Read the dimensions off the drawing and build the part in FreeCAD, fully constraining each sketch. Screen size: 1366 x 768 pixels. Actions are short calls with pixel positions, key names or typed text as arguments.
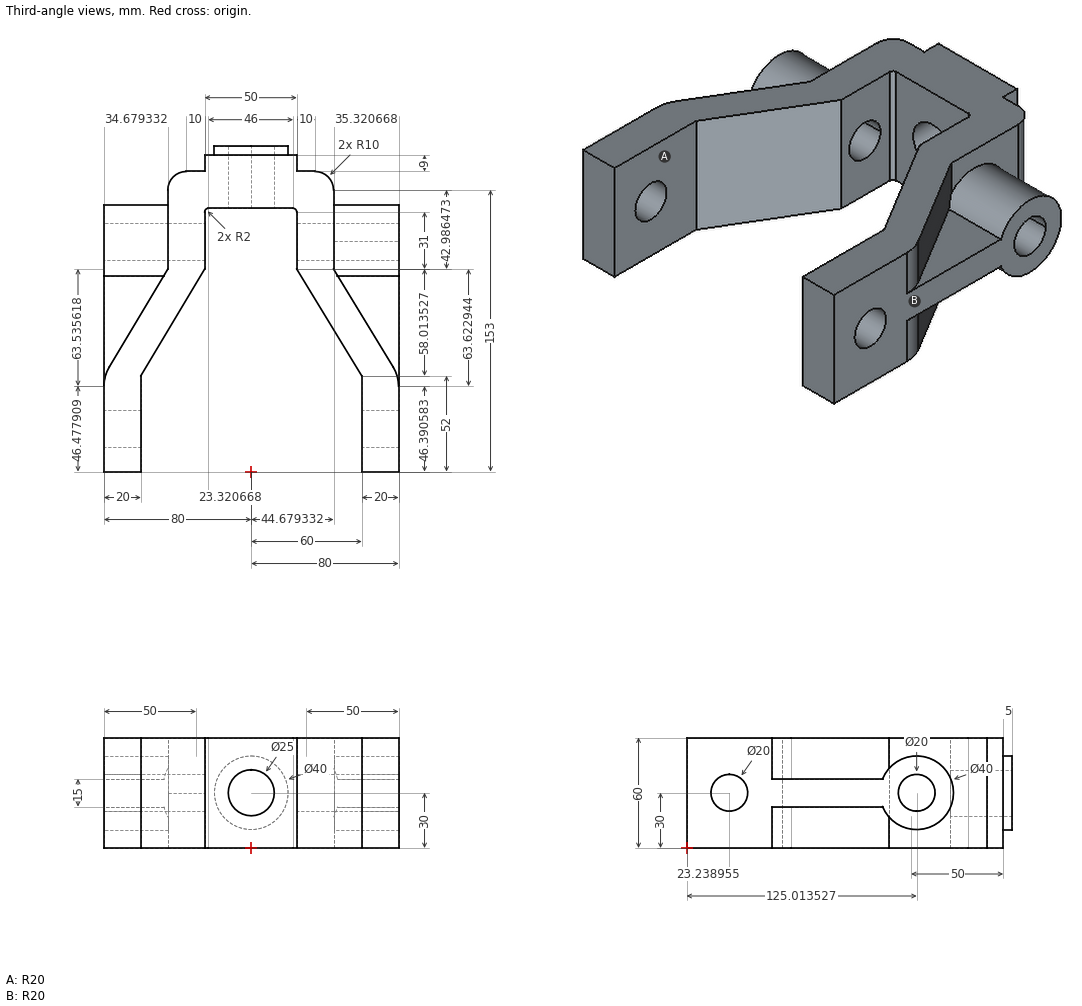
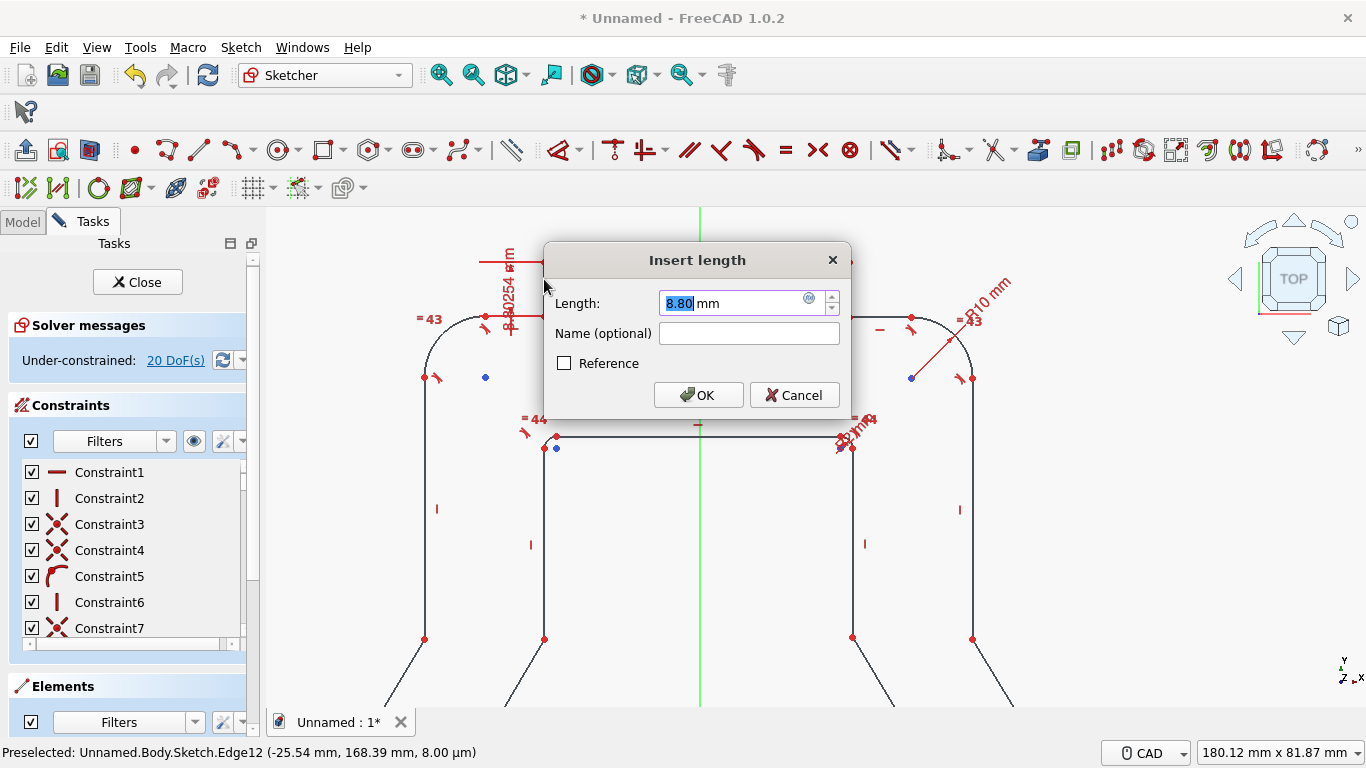
text(9)
key(Return)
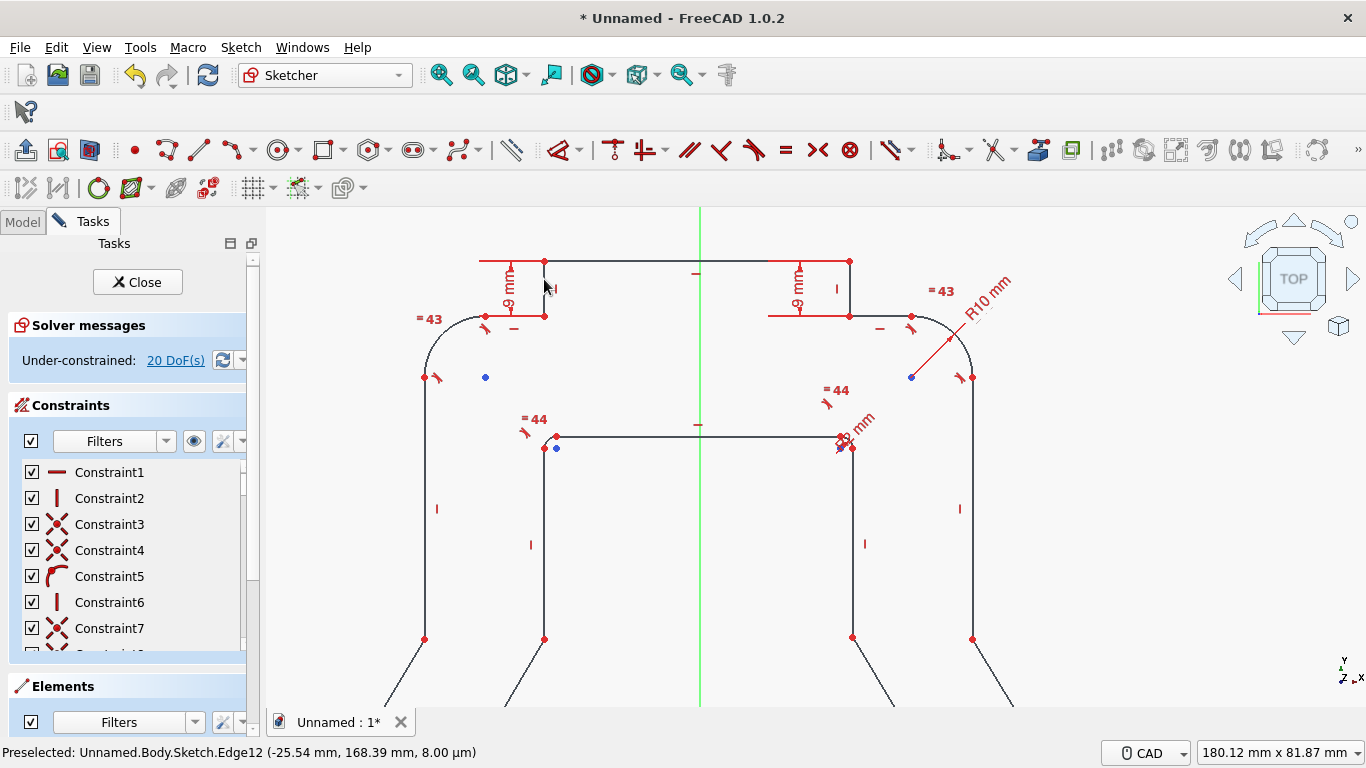
click(642, 437)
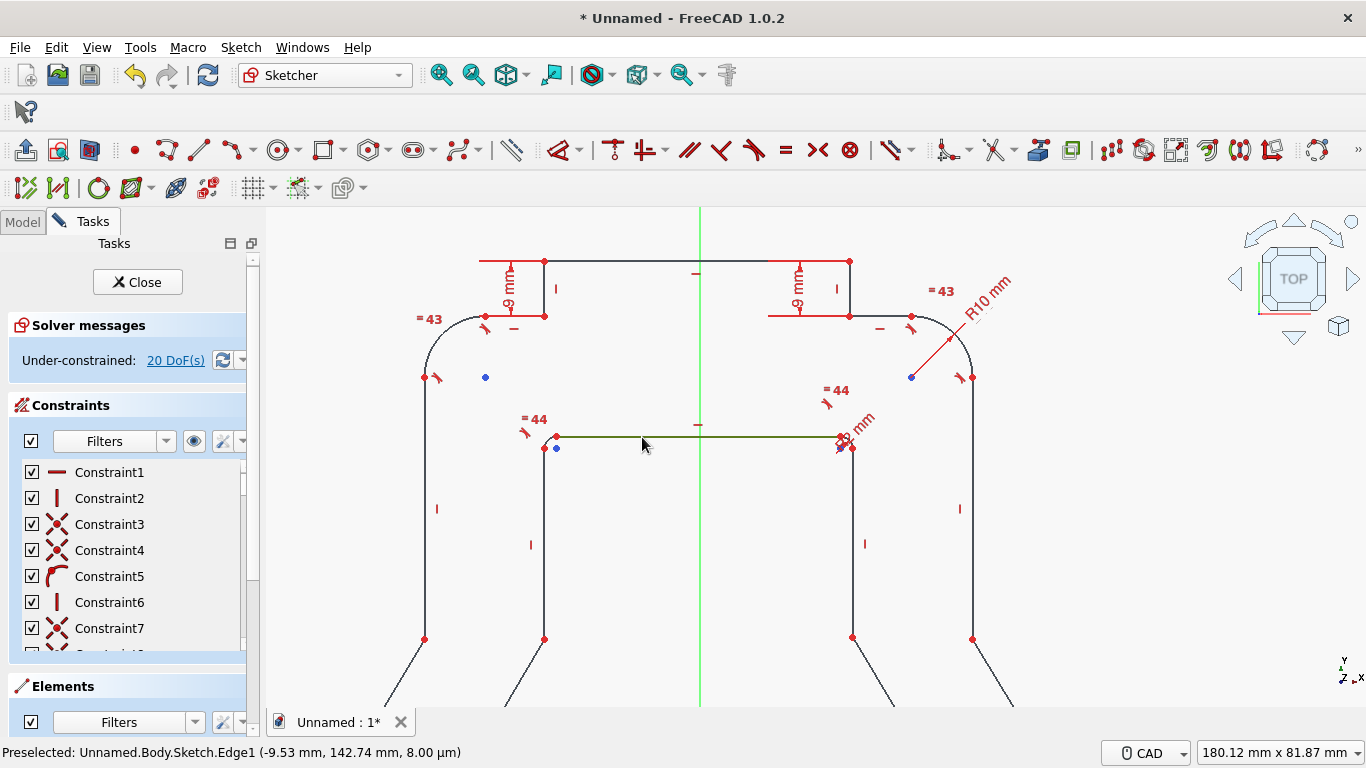
key(l)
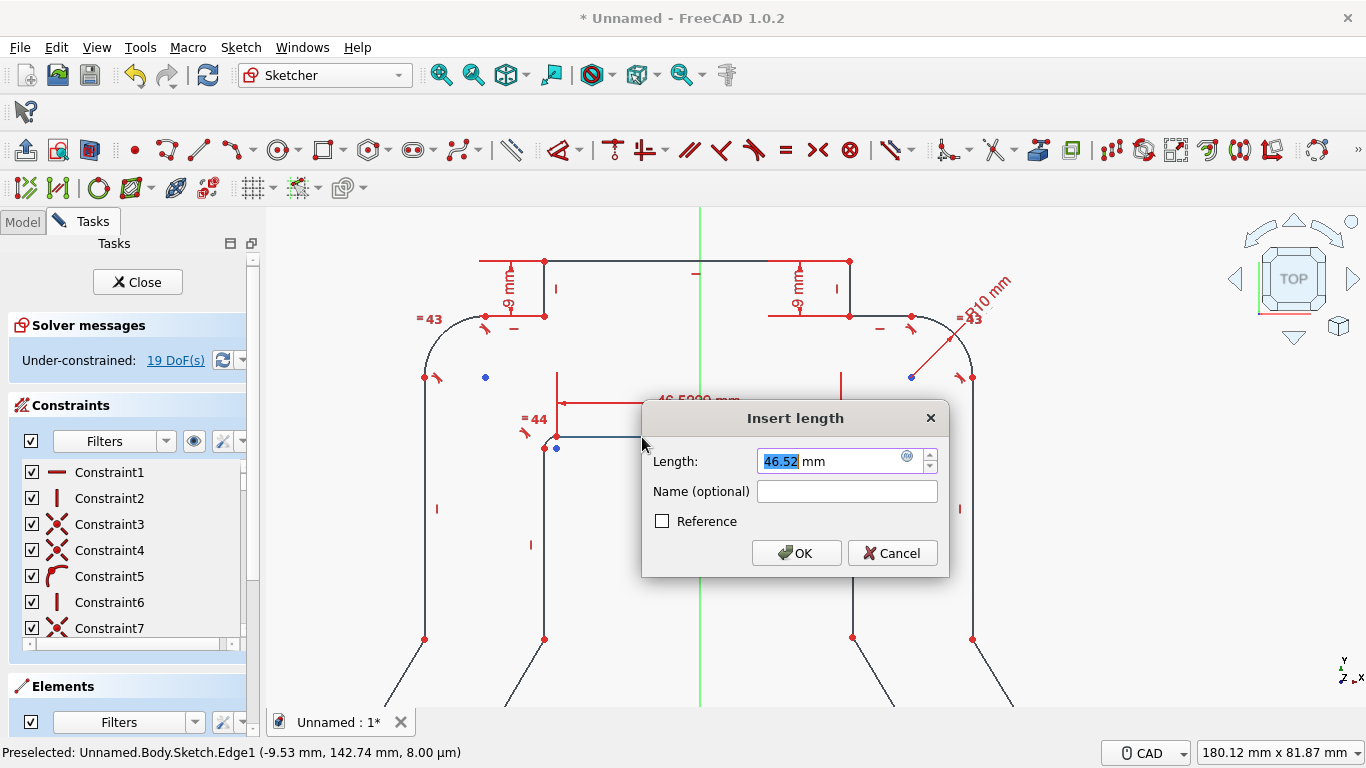
text(46)
key(Return)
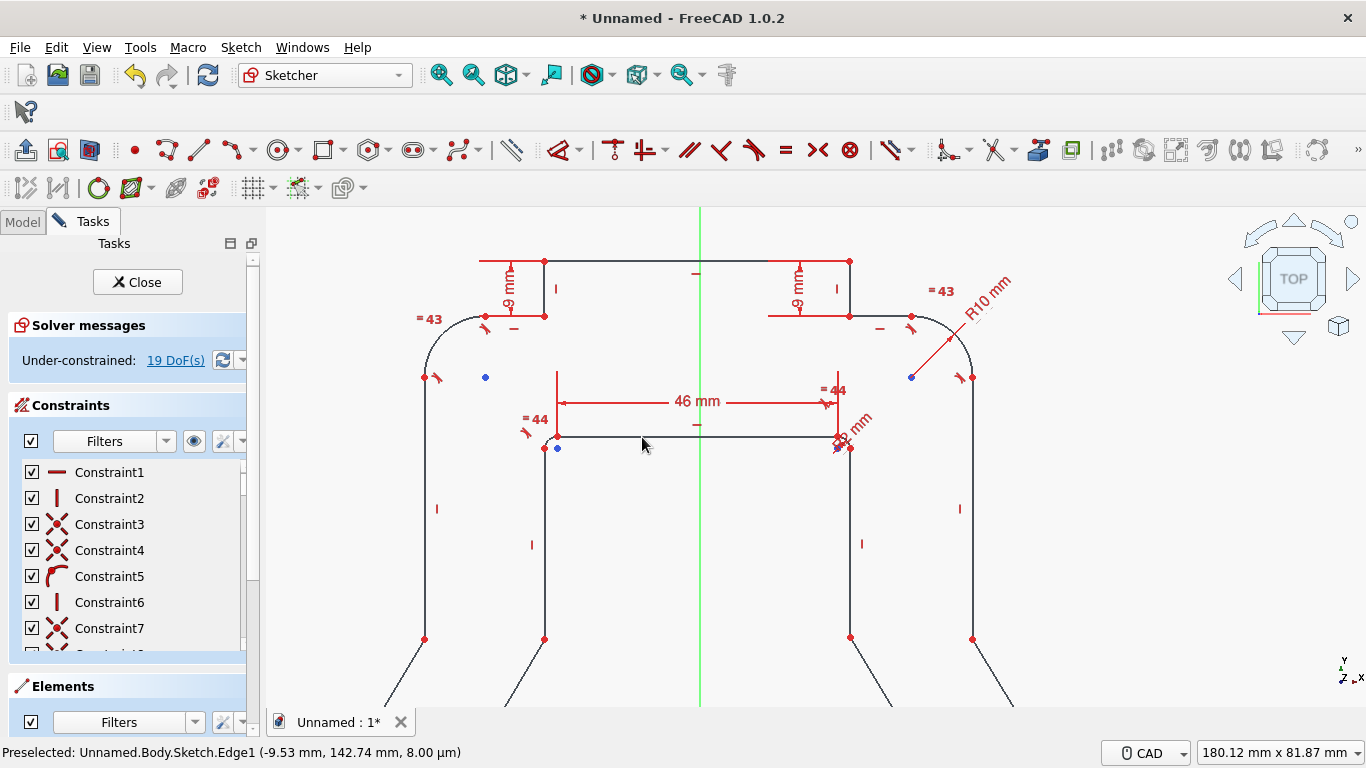
click(850, 505)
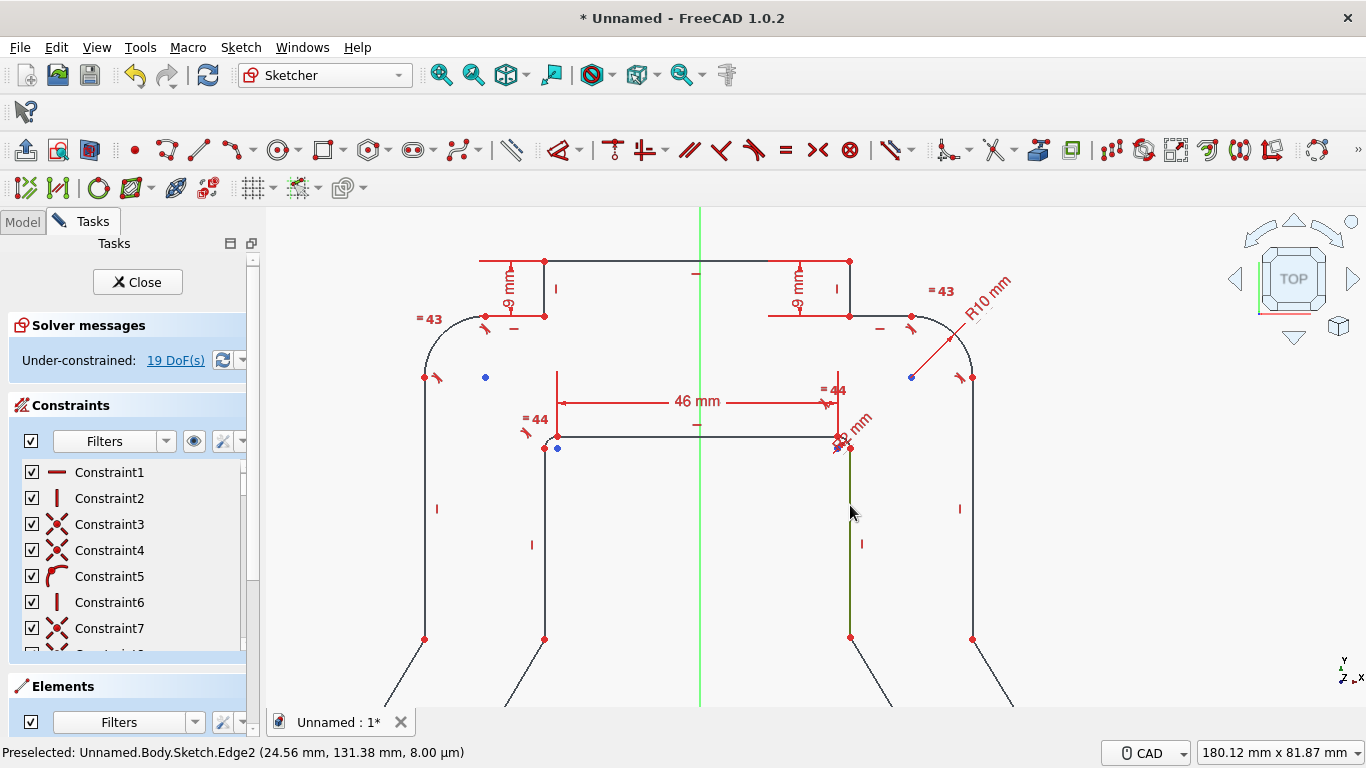
key(i)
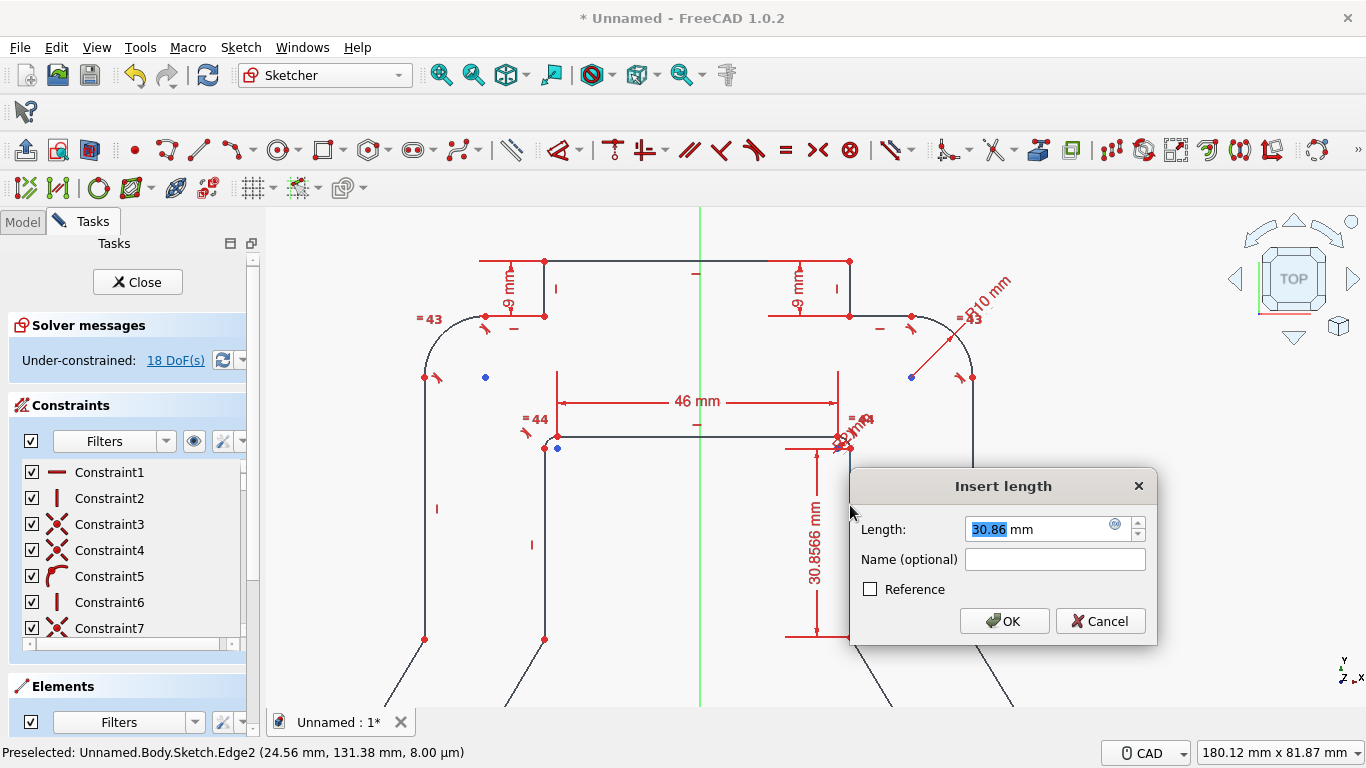
text(31)
key(Return)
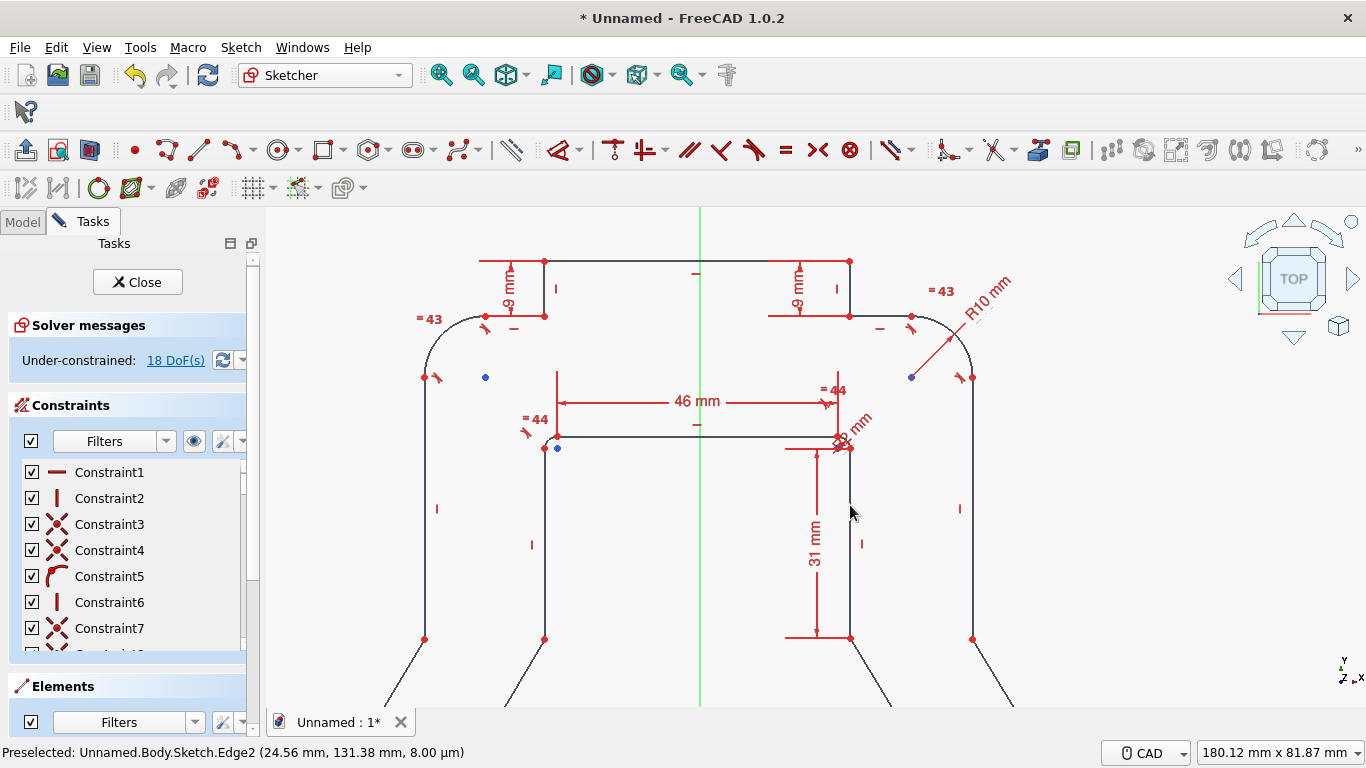
scroll(768, 316, down, 6)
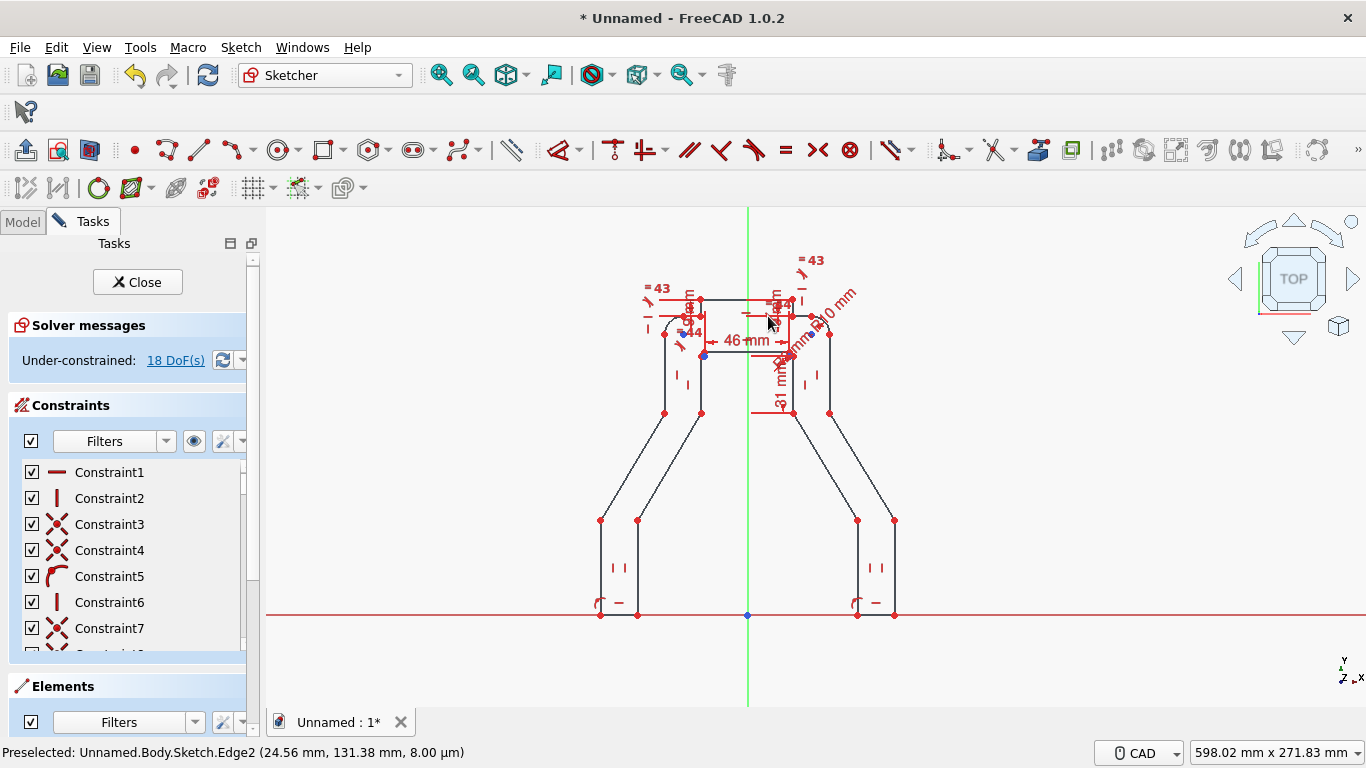
click(858, 549)